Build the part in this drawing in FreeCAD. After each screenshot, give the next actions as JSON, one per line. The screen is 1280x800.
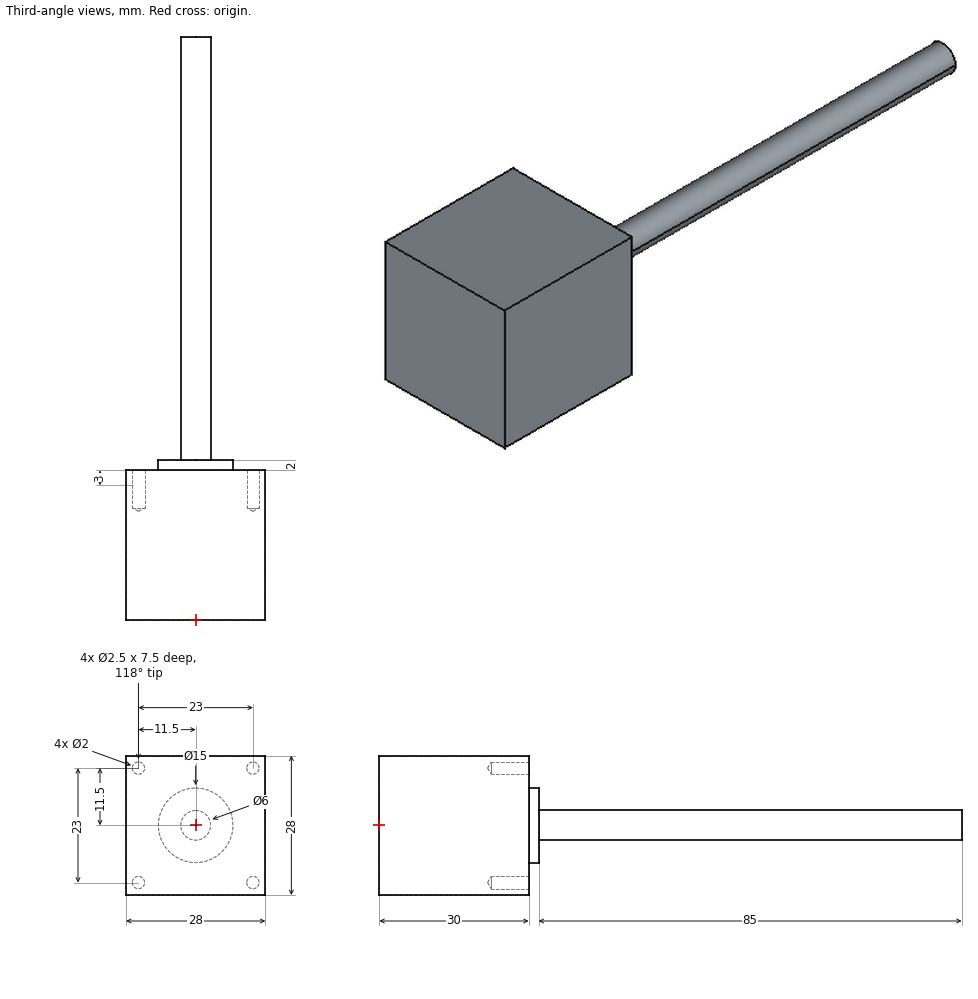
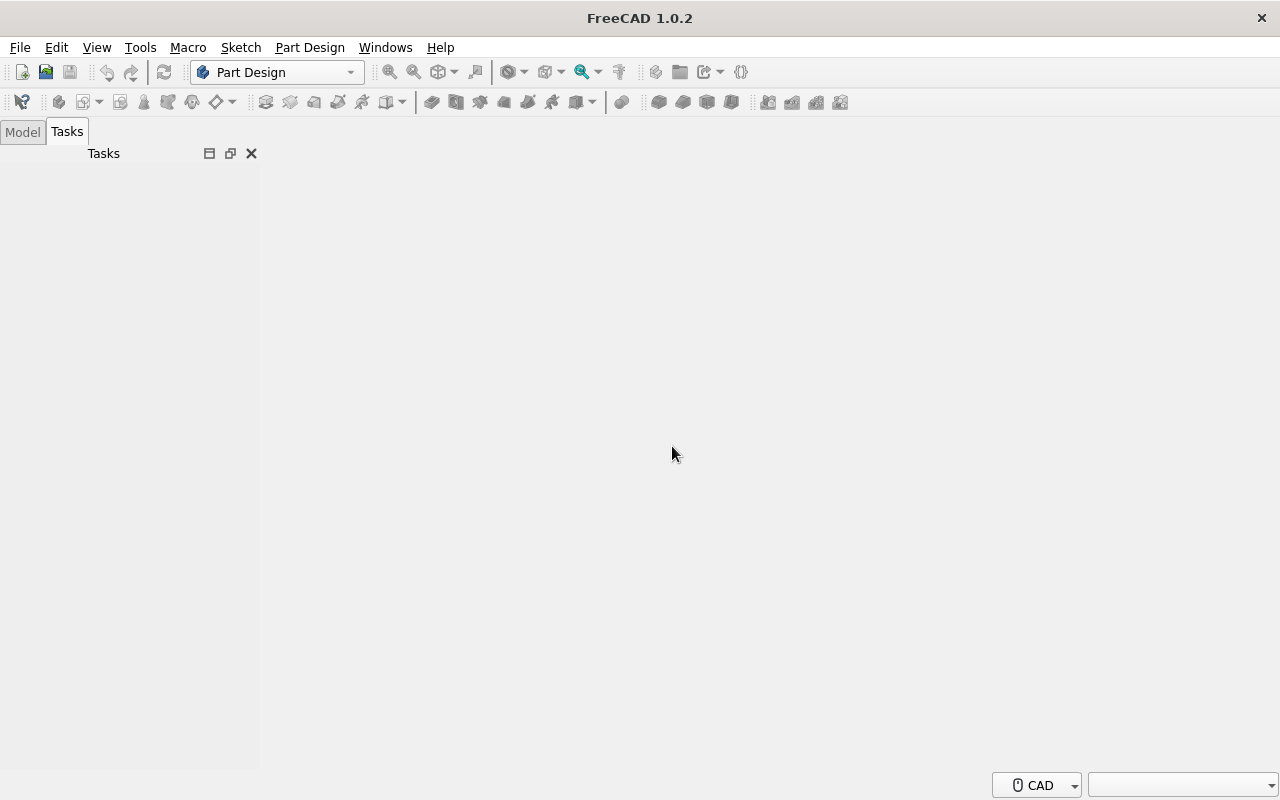
{"action": "left_click", "coordinate": [22, 72]}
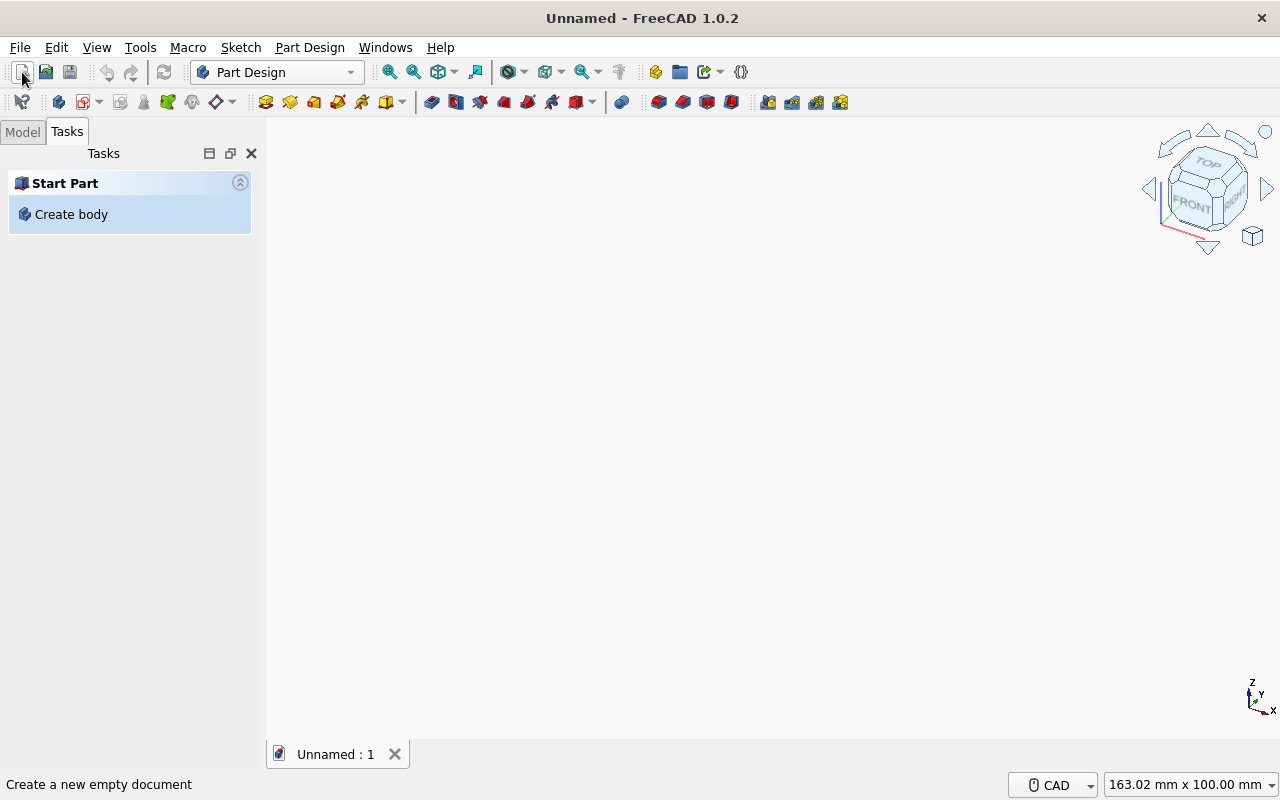
{"action": "left_click", "coordinate": [84, 102]}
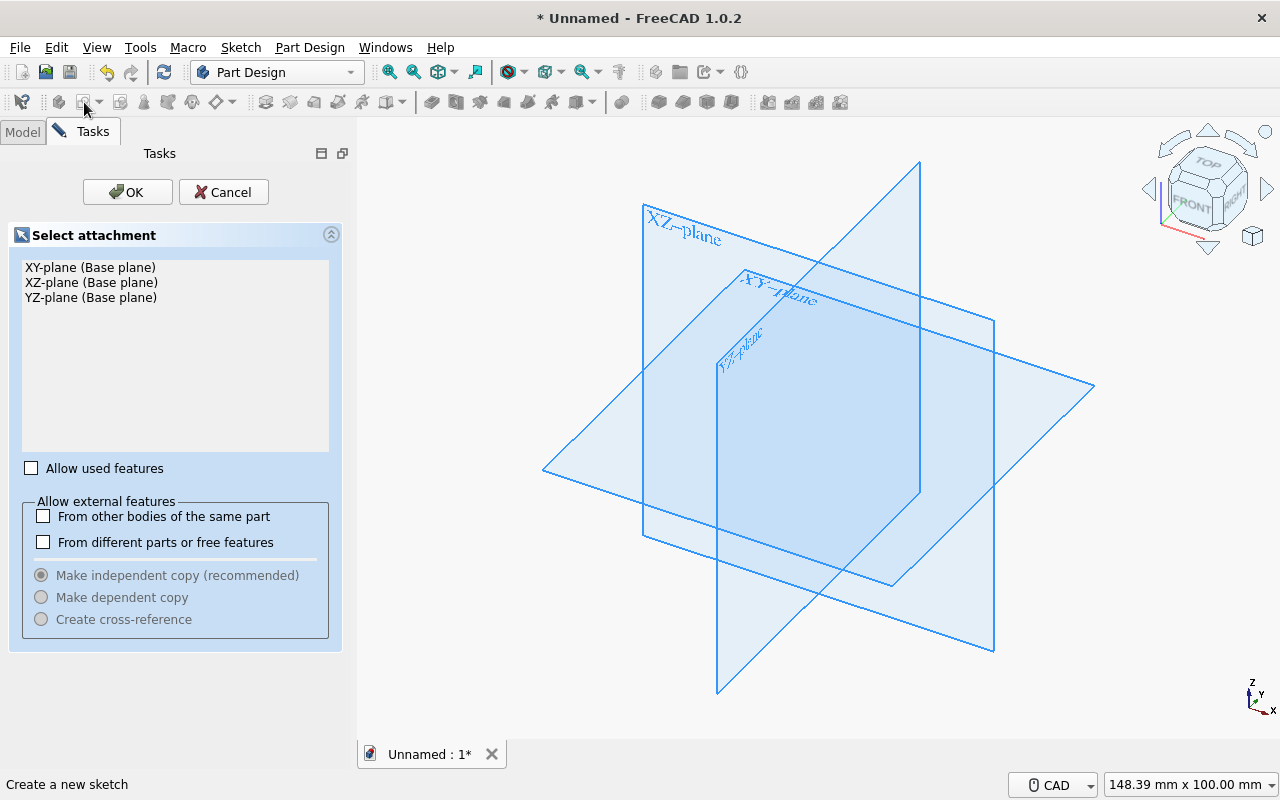
{"action": "left_click", "coordinate": [82, 282]}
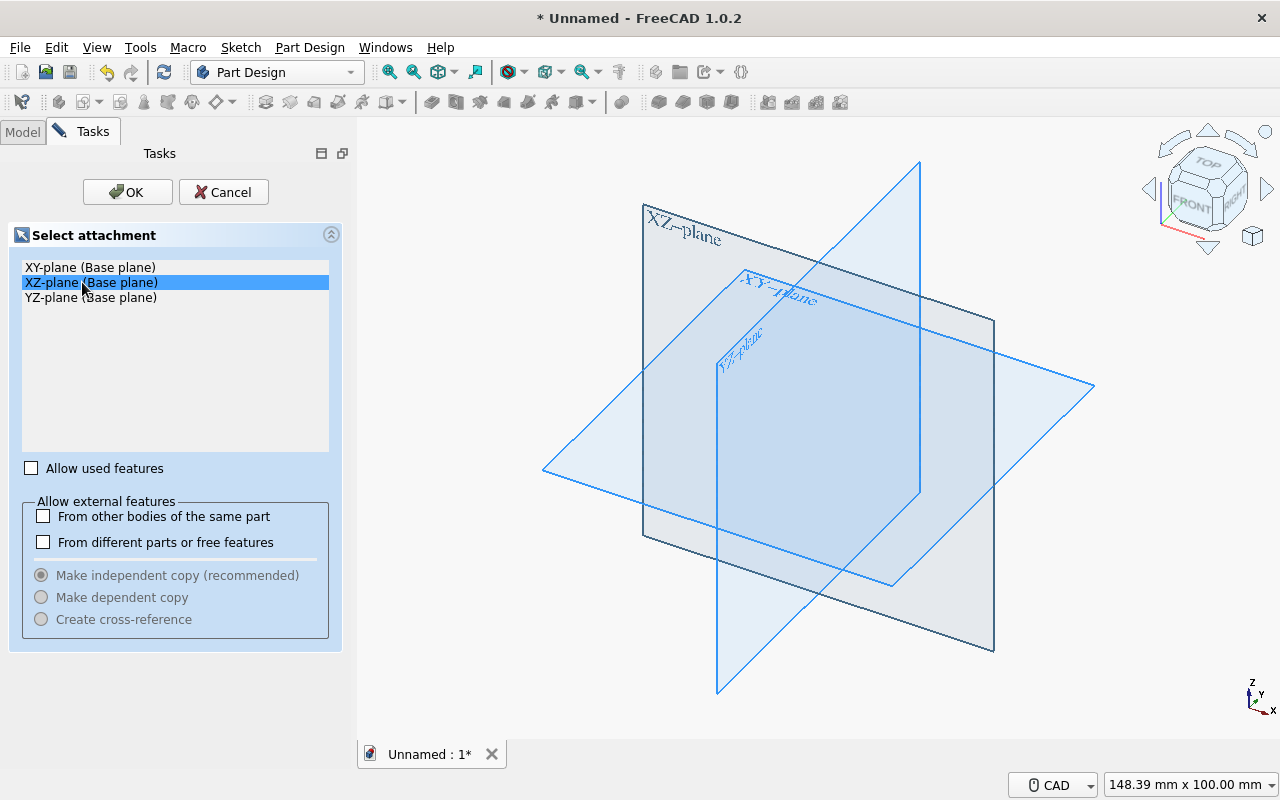
{"action": "left_click", "coordinate": [128, 192]}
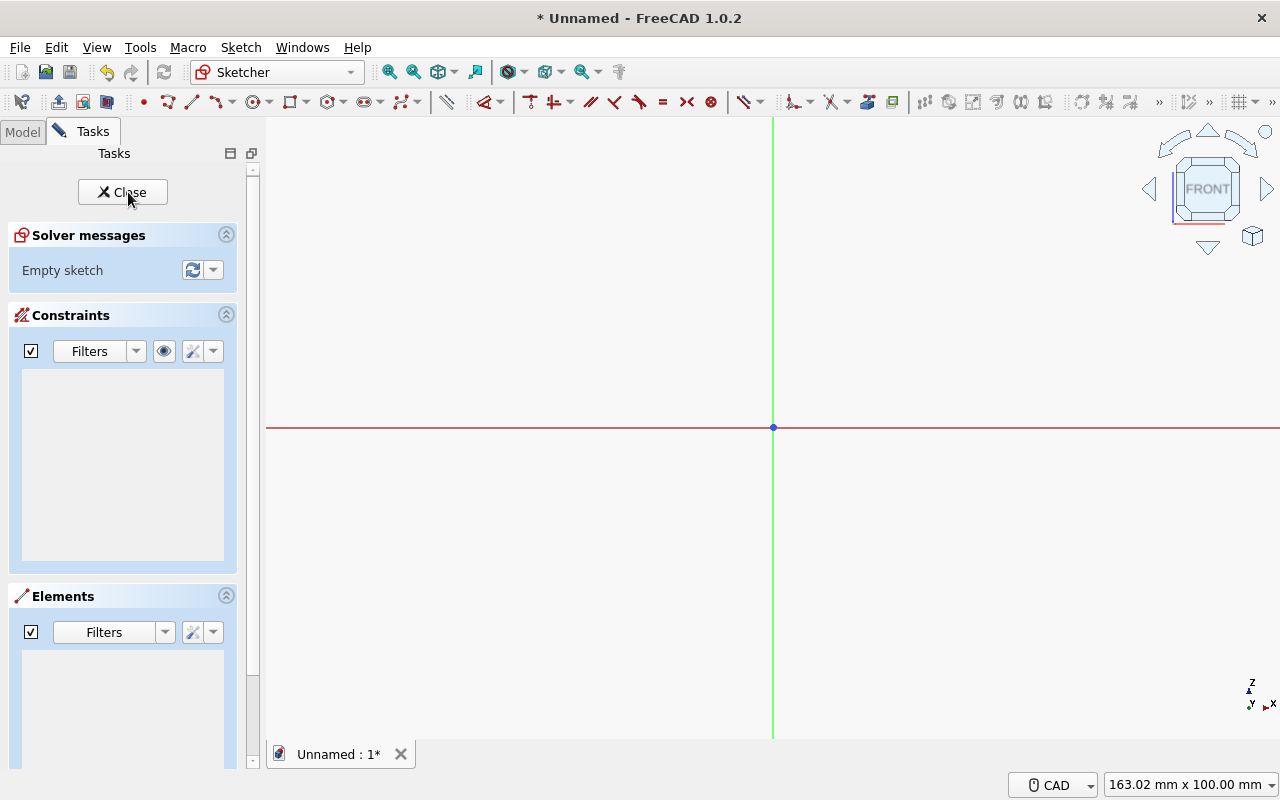
{"action": "scroll", "coordinate": [829, 428], "scroll_direction": "up", "scroll_amount": 4}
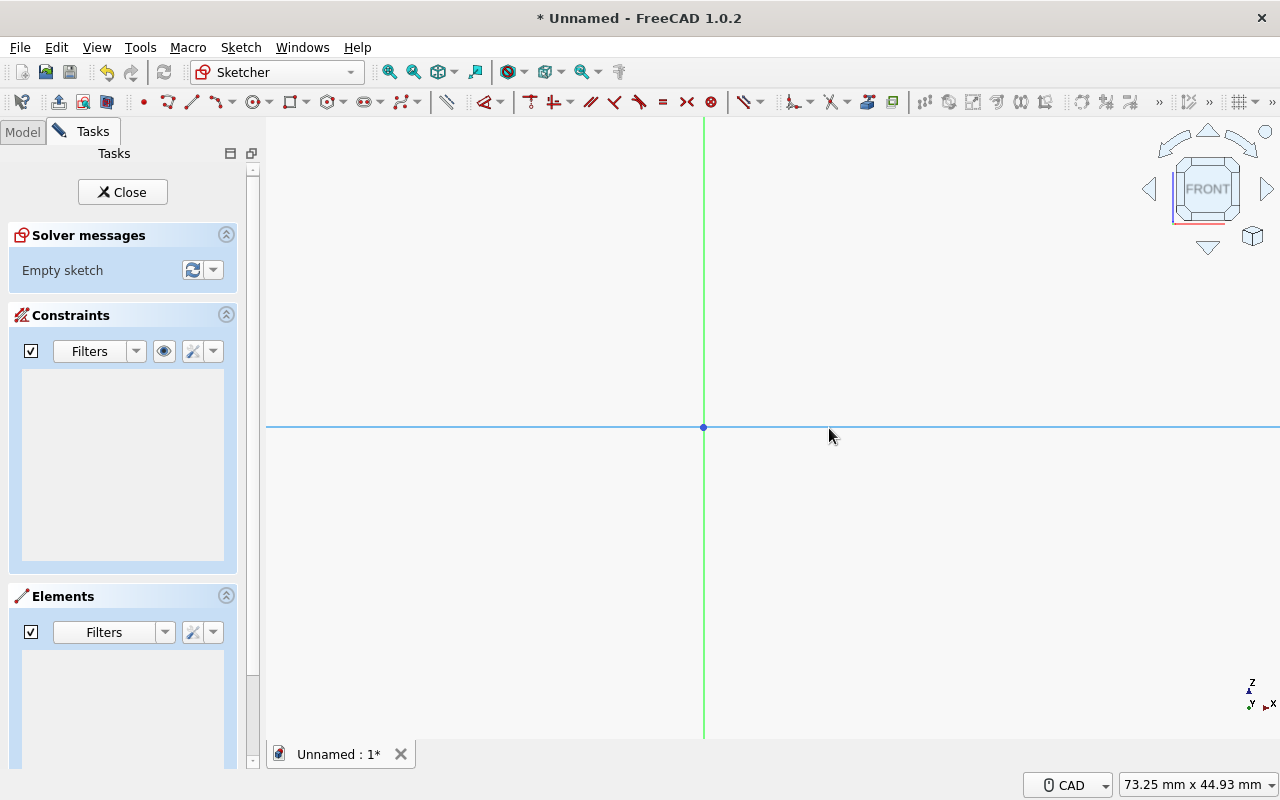
{"action": "key", "text": "g v"}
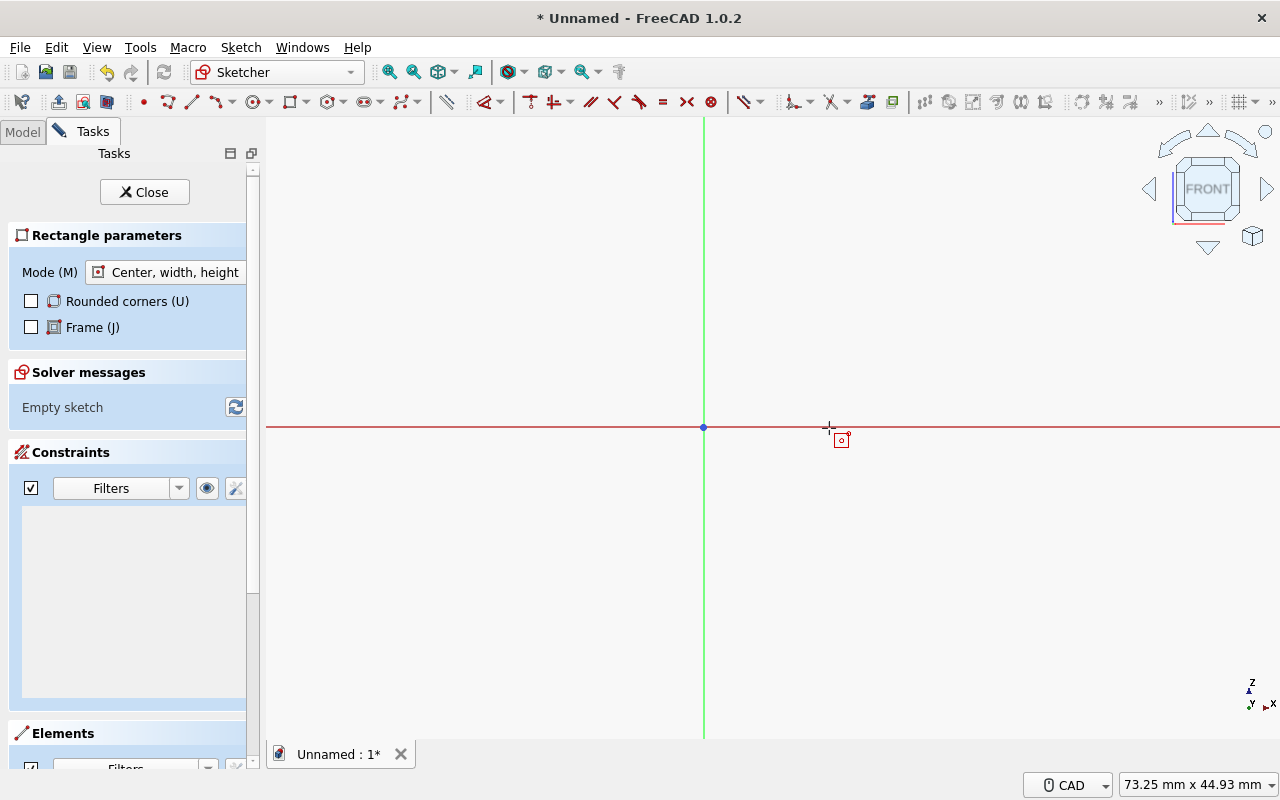
{"action": "left_click", "coordinate": [704, 427]}
{"action": "left_click", "coordinate": [897, 234]}
{"action": "key", "text": "Escape"}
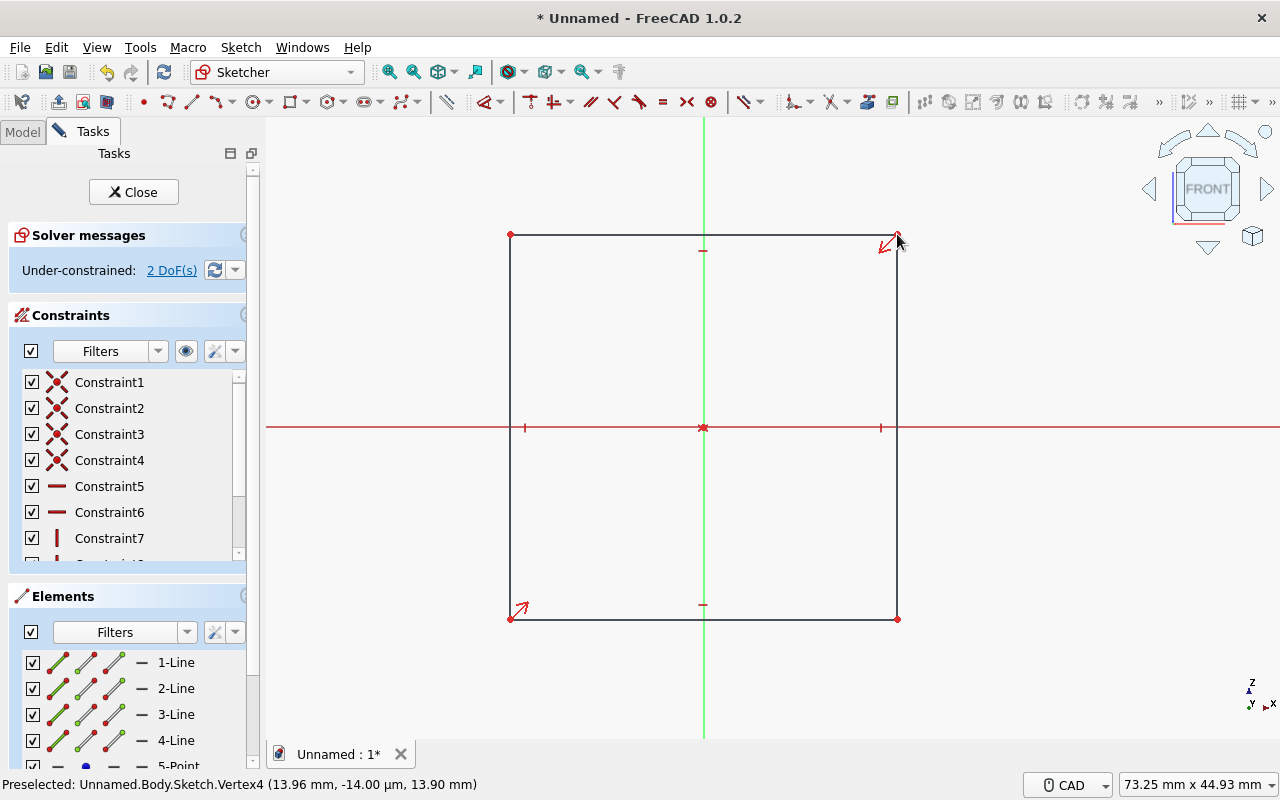
{"action": "left_click", "coordinate": [484, 102]}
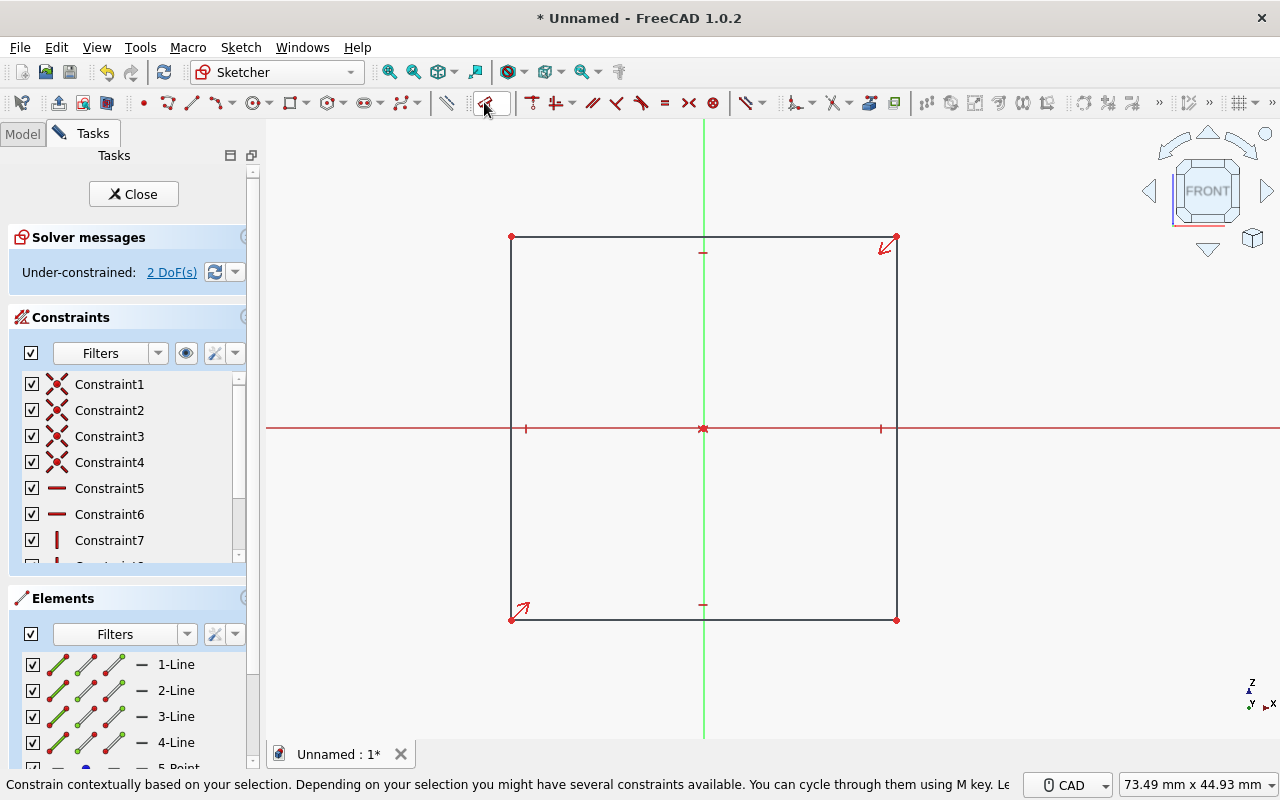
{"action": "left_click", "coordinate": [627, 620]}
{"action": "left_click", "coordinate": [615, 654]}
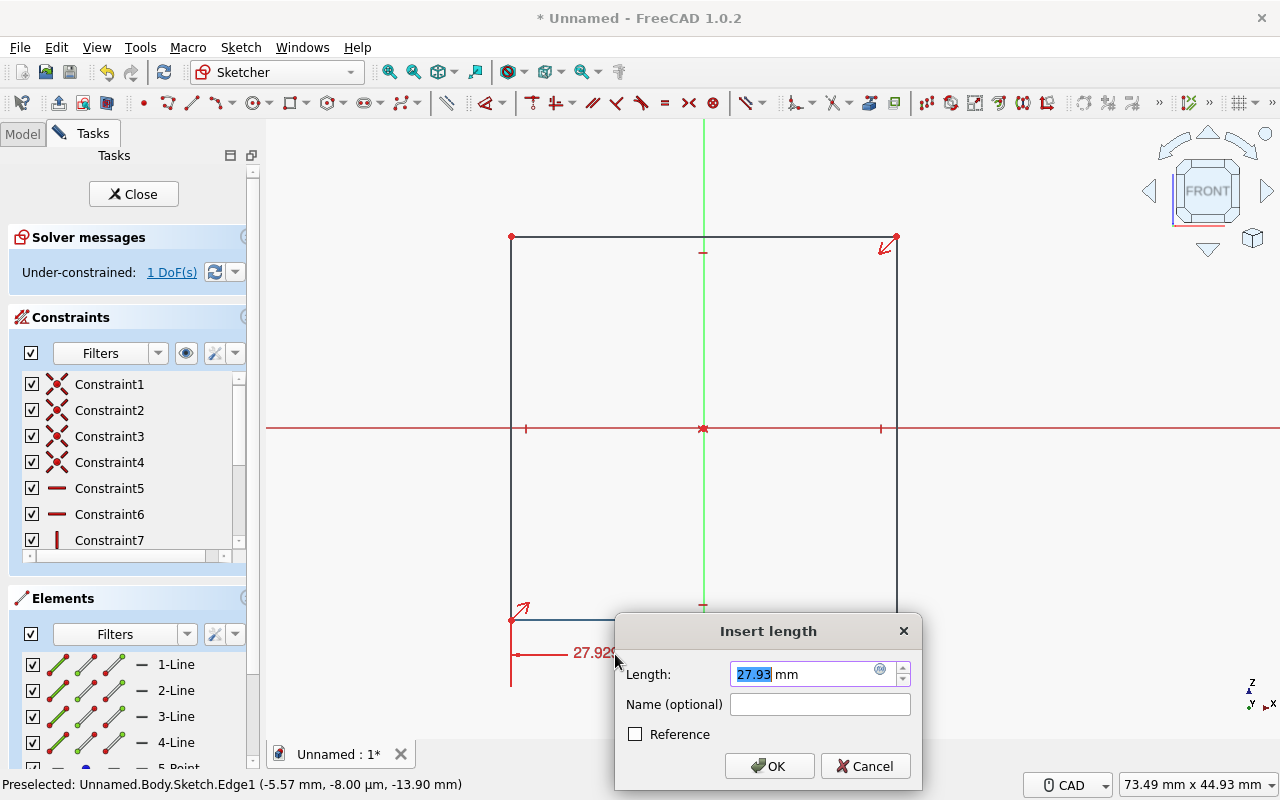
{"action": "type", "text": "28"}
{"action": "key", "text": "Return"}